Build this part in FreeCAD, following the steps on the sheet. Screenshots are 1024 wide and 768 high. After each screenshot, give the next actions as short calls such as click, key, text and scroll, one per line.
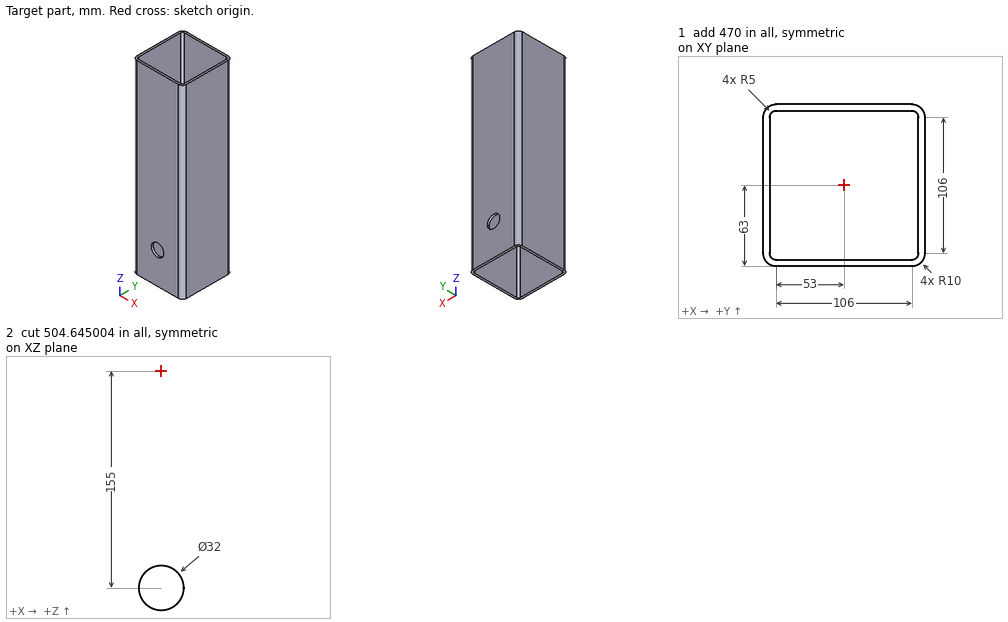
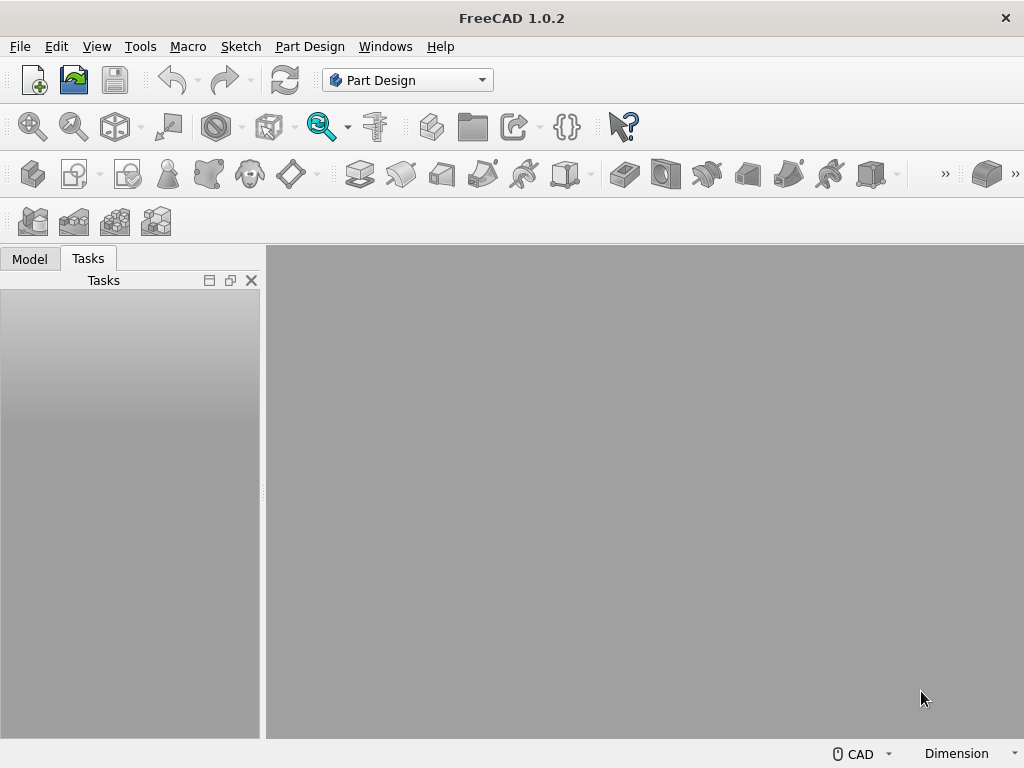
click(33, 80)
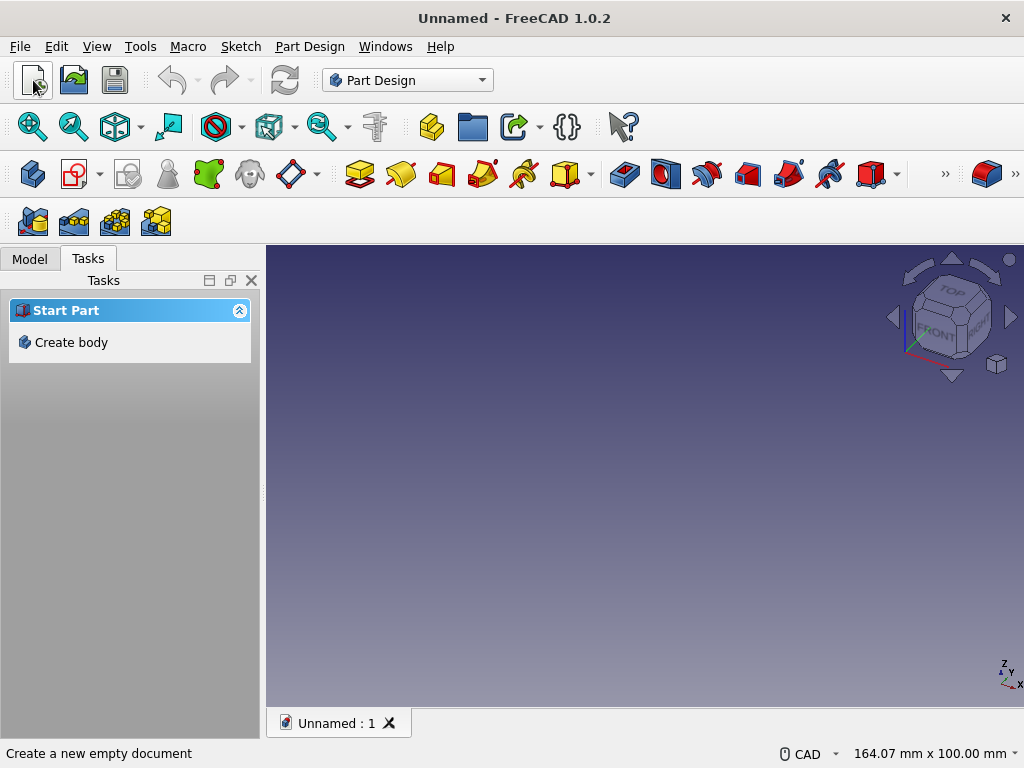
click(74, 174)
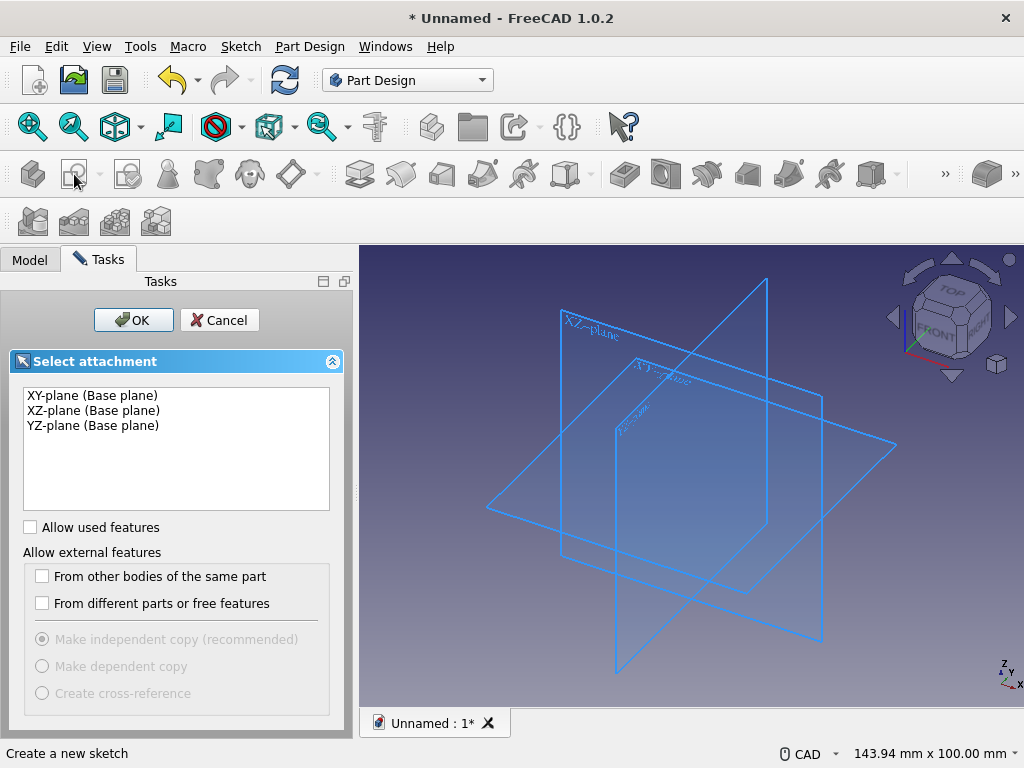
click(84, 396)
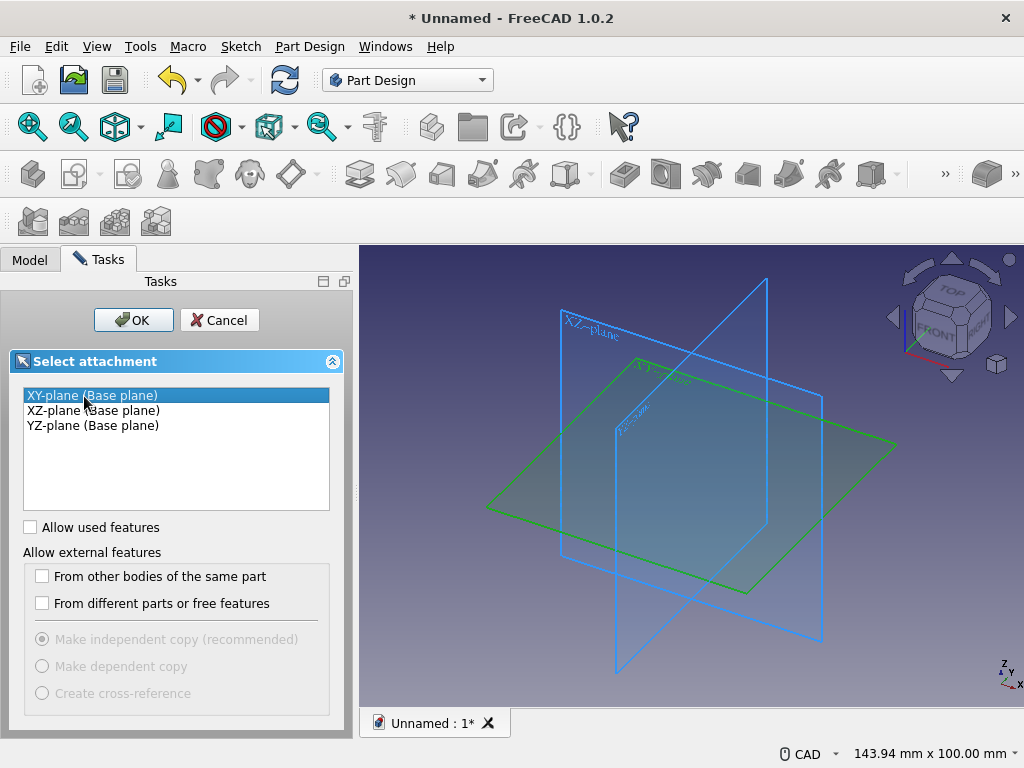
click(134, 320)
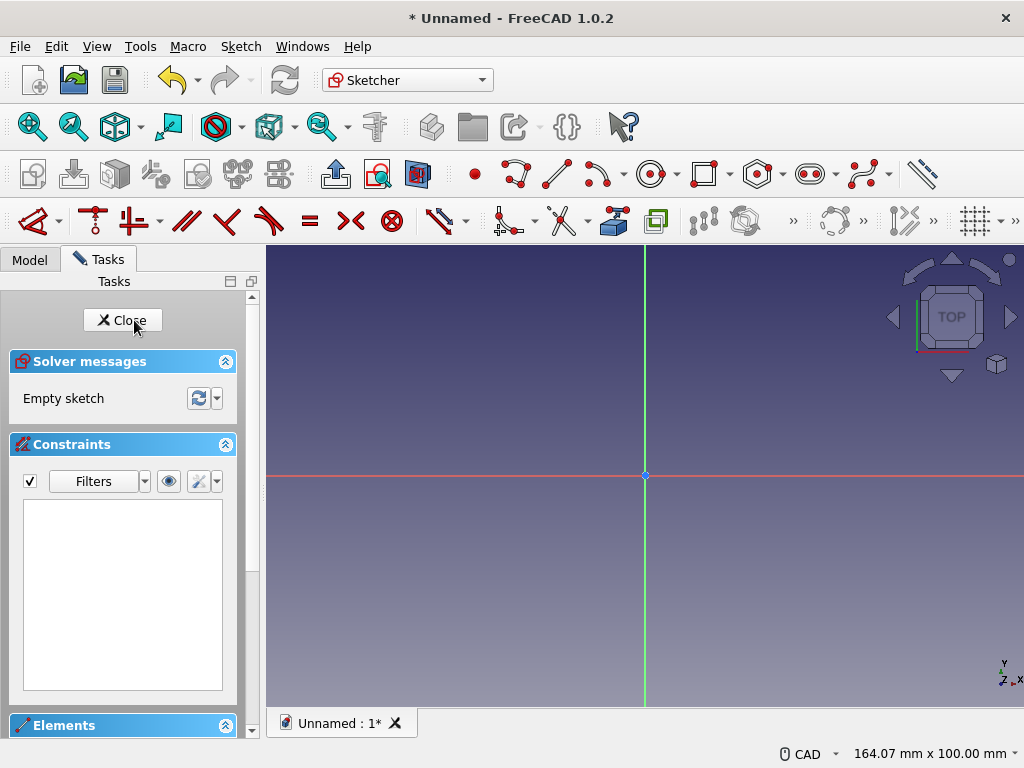
scroll(521, 476, down, 4)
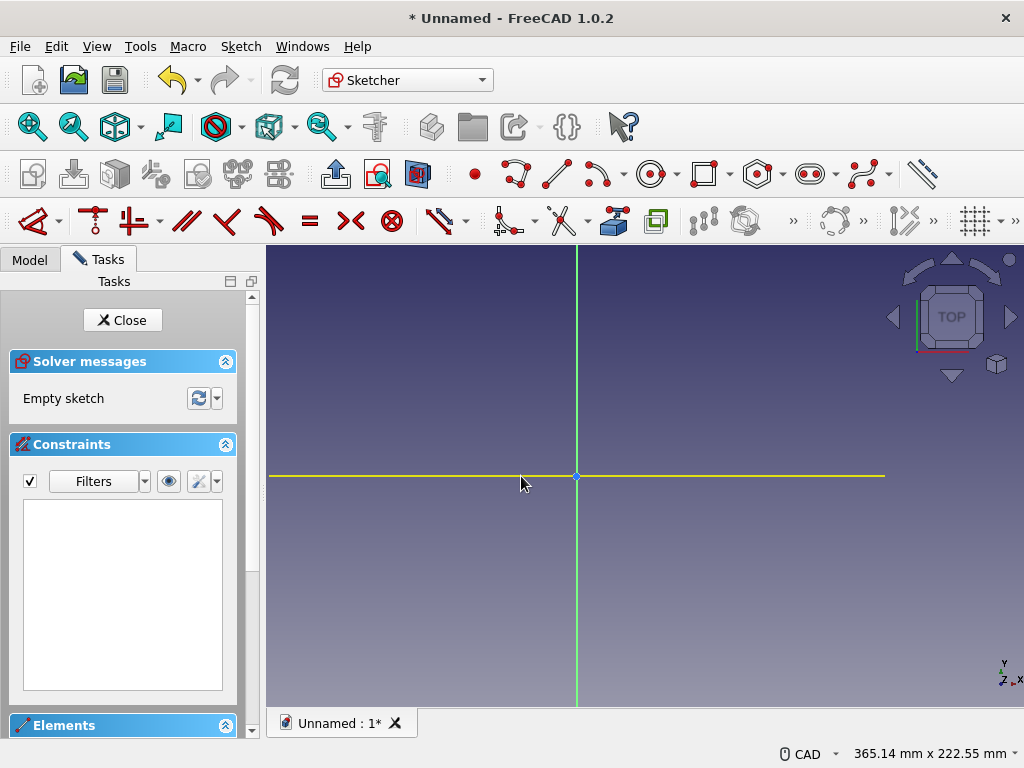
click(557, 174)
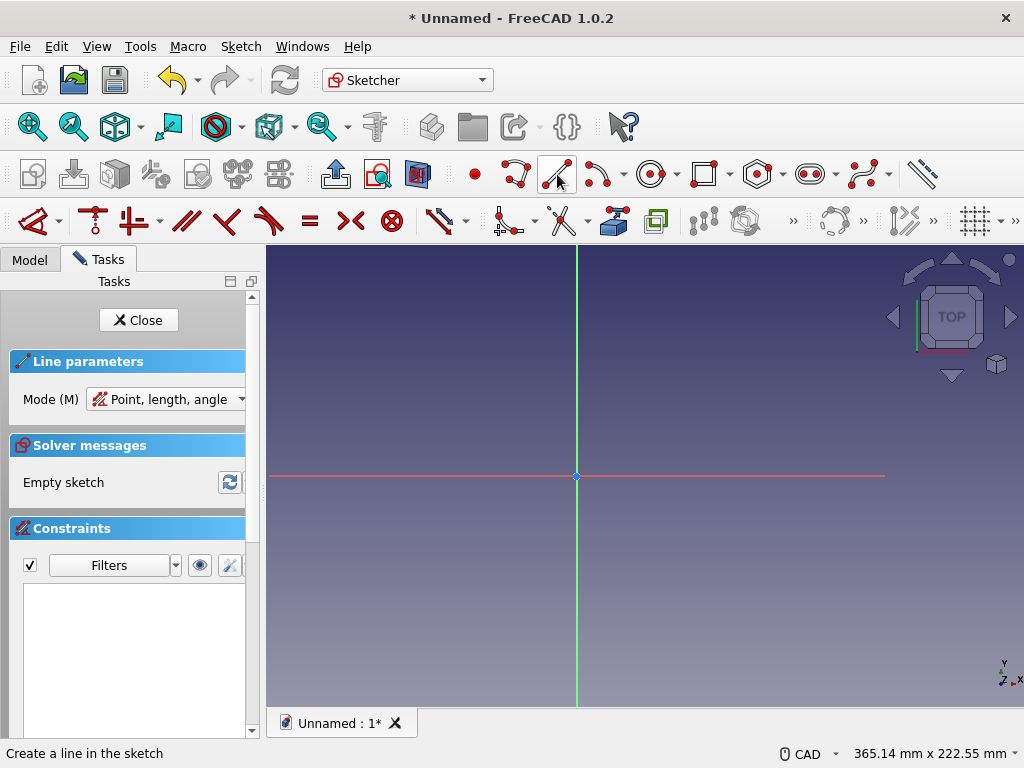
click(467, 607)
click(687, 607)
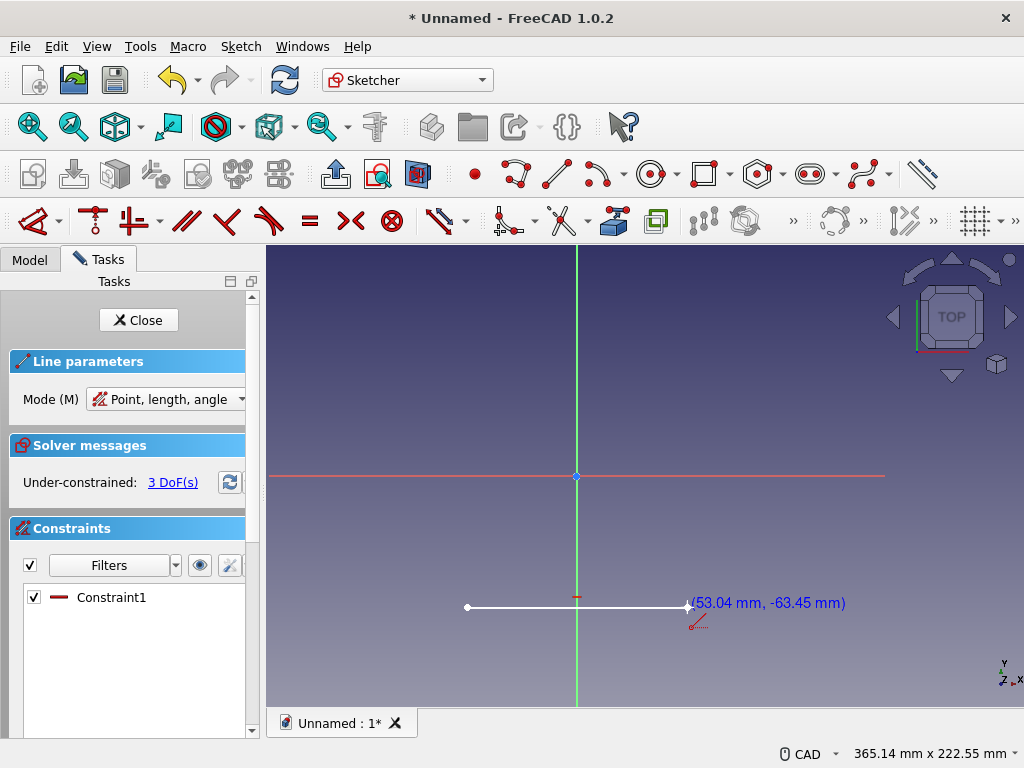
click(708, 586)
click(708, 366)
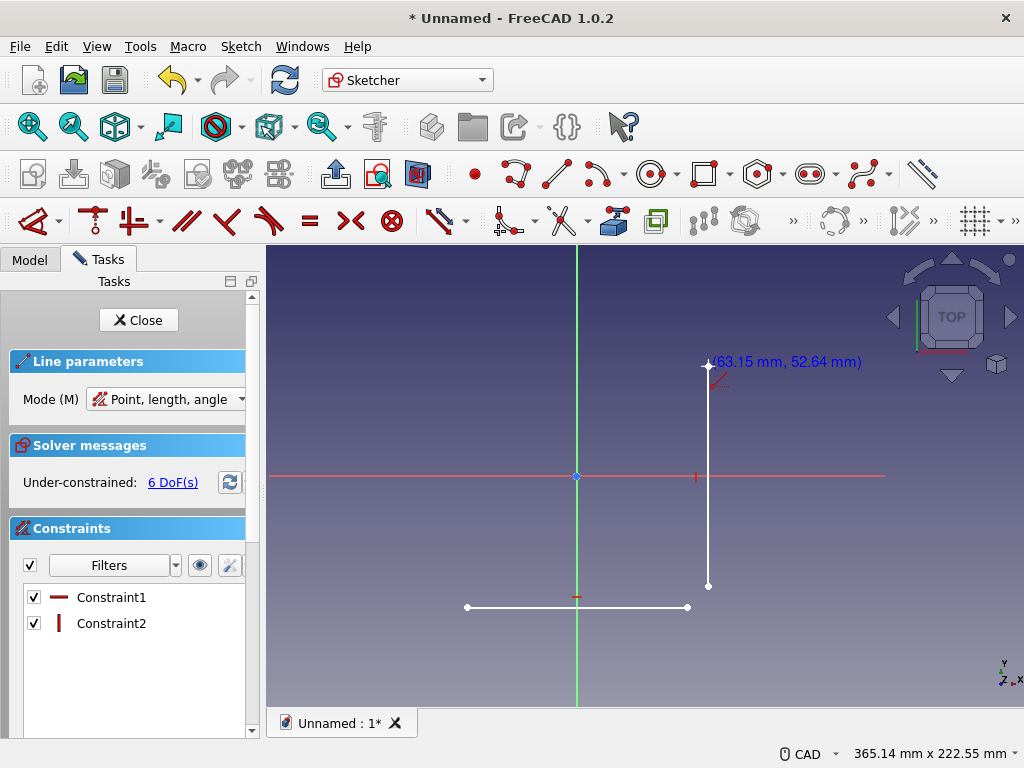
click(687, 345)
click(467, 345)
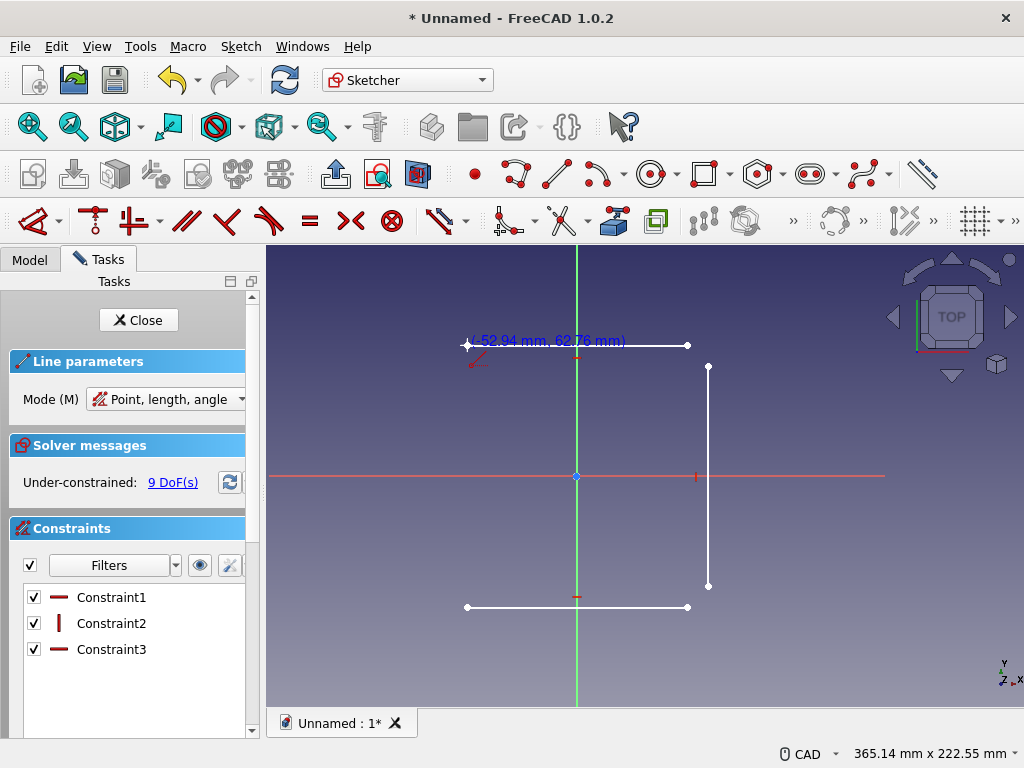
click(446, 366)
click(446, 586)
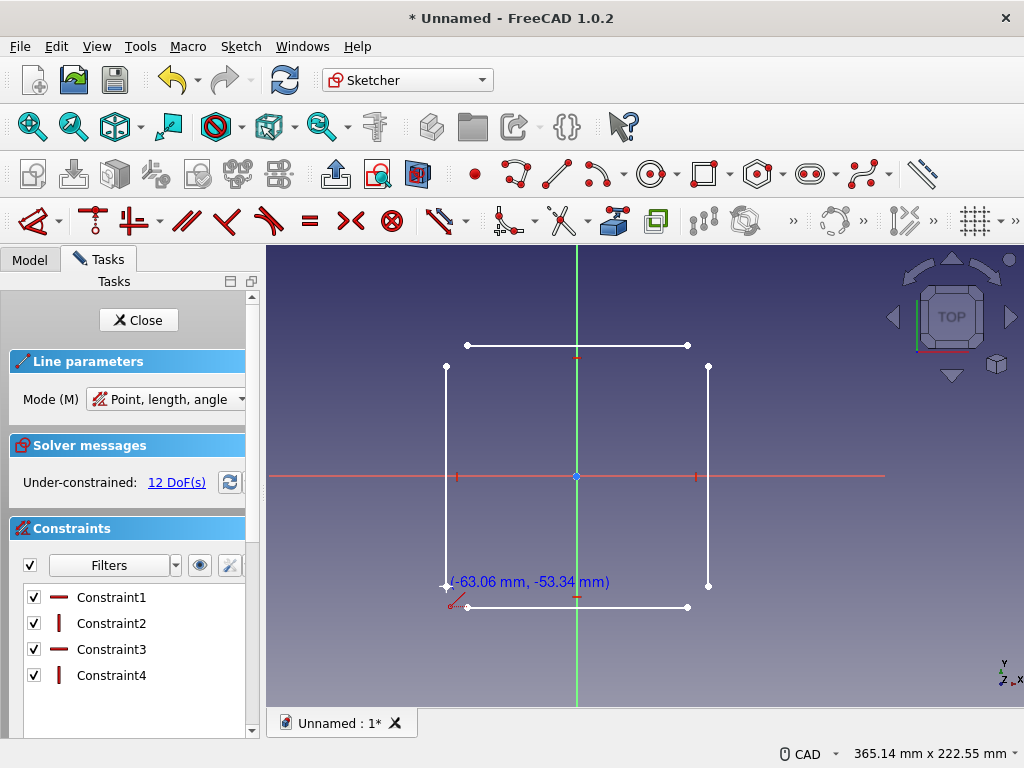
click(624, 174)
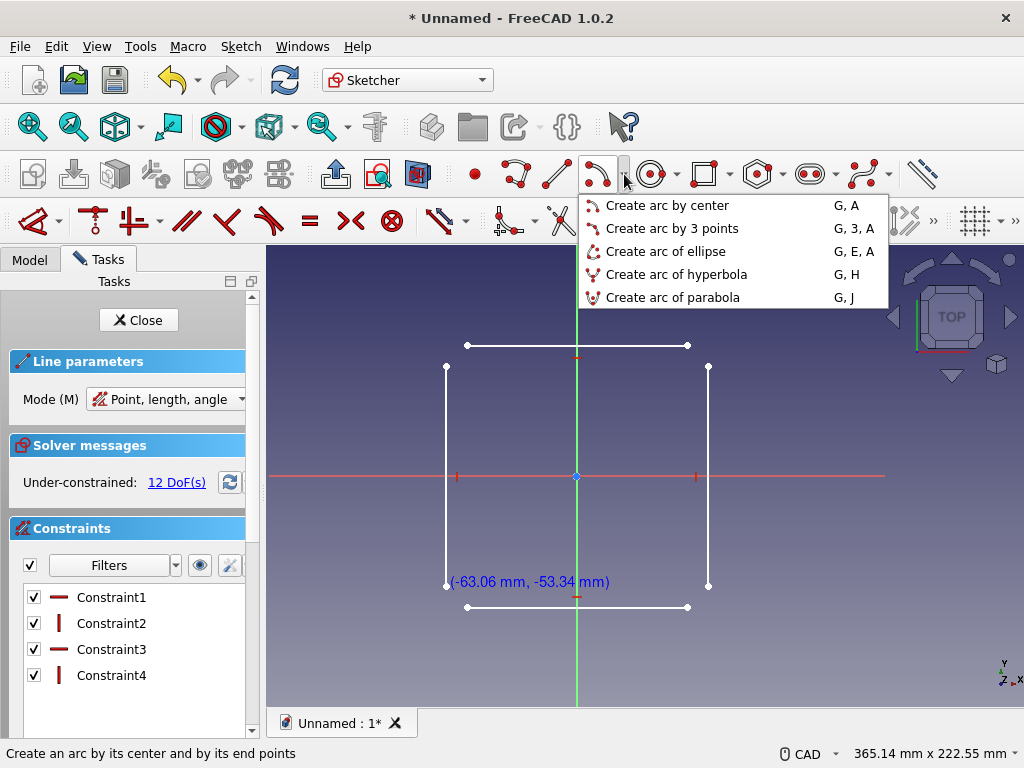
click(734, 228)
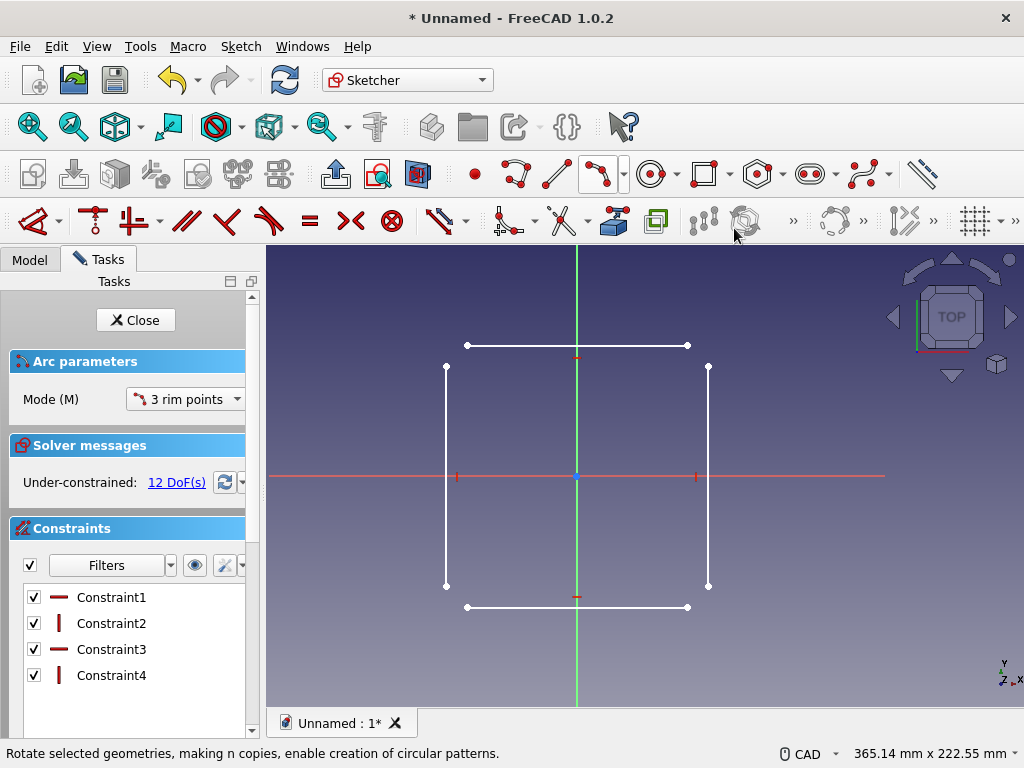
click(687, 608)
click(708, 587)